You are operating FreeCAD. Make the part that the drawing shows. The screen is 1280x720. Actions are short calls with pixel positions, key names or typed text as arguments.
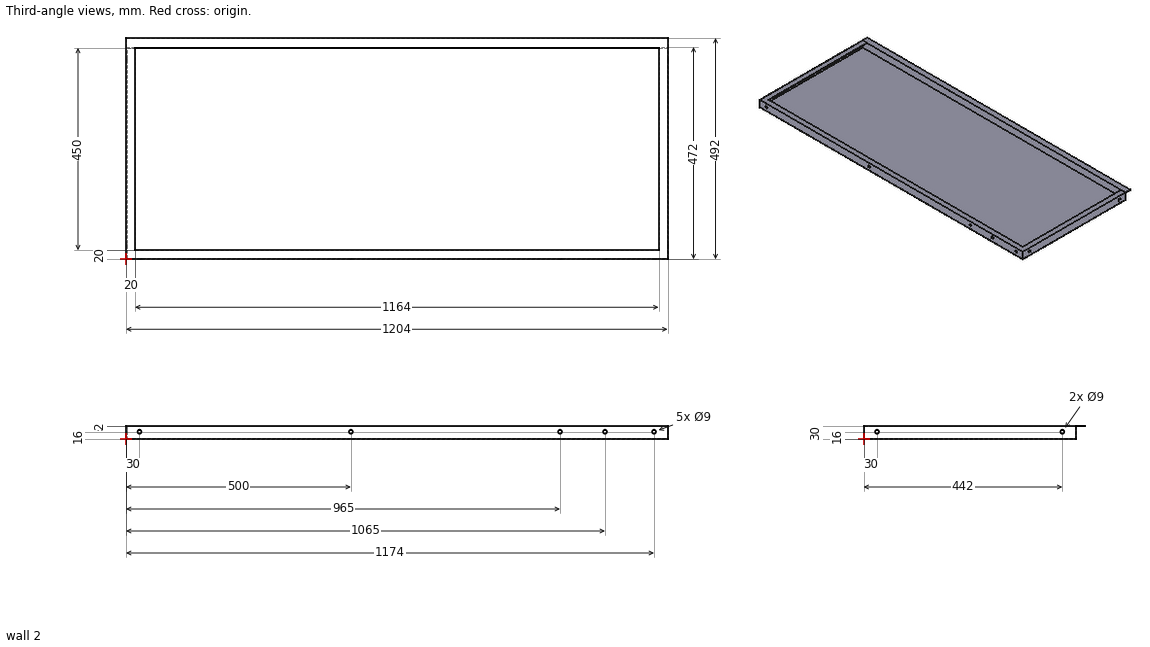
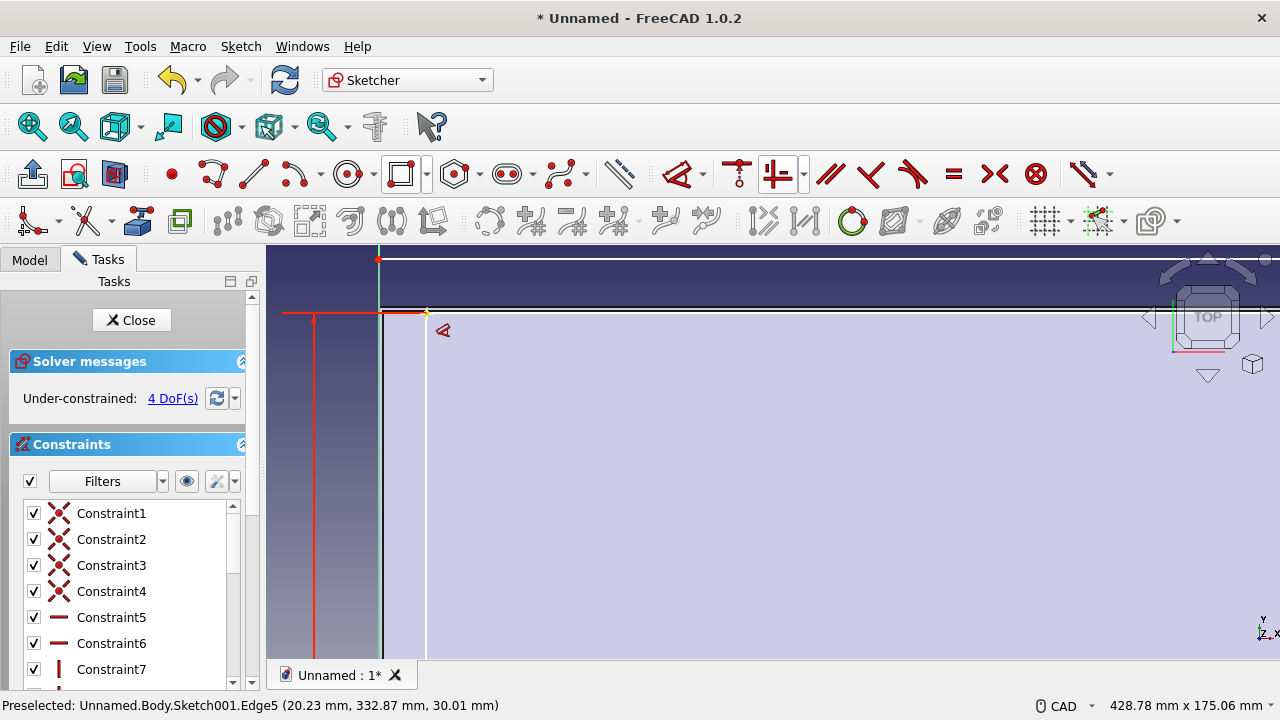
click(426, 313)
click(403, 279)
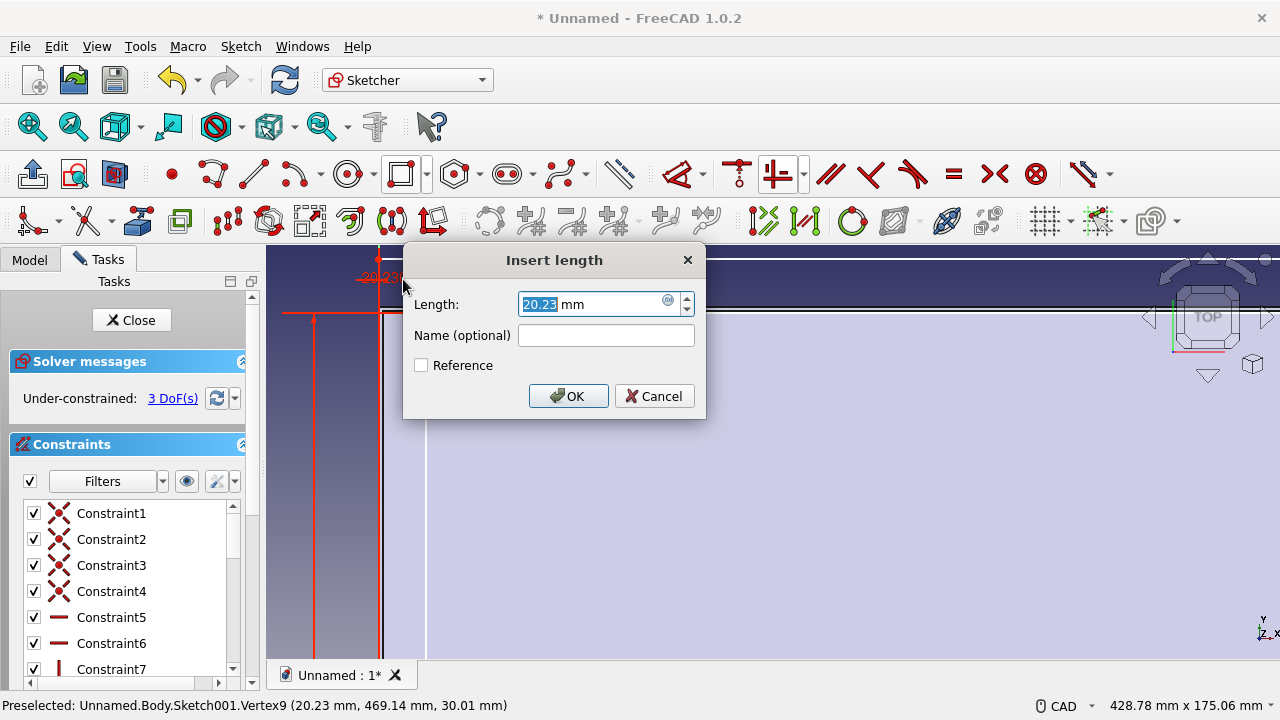
text(20)
key(Return)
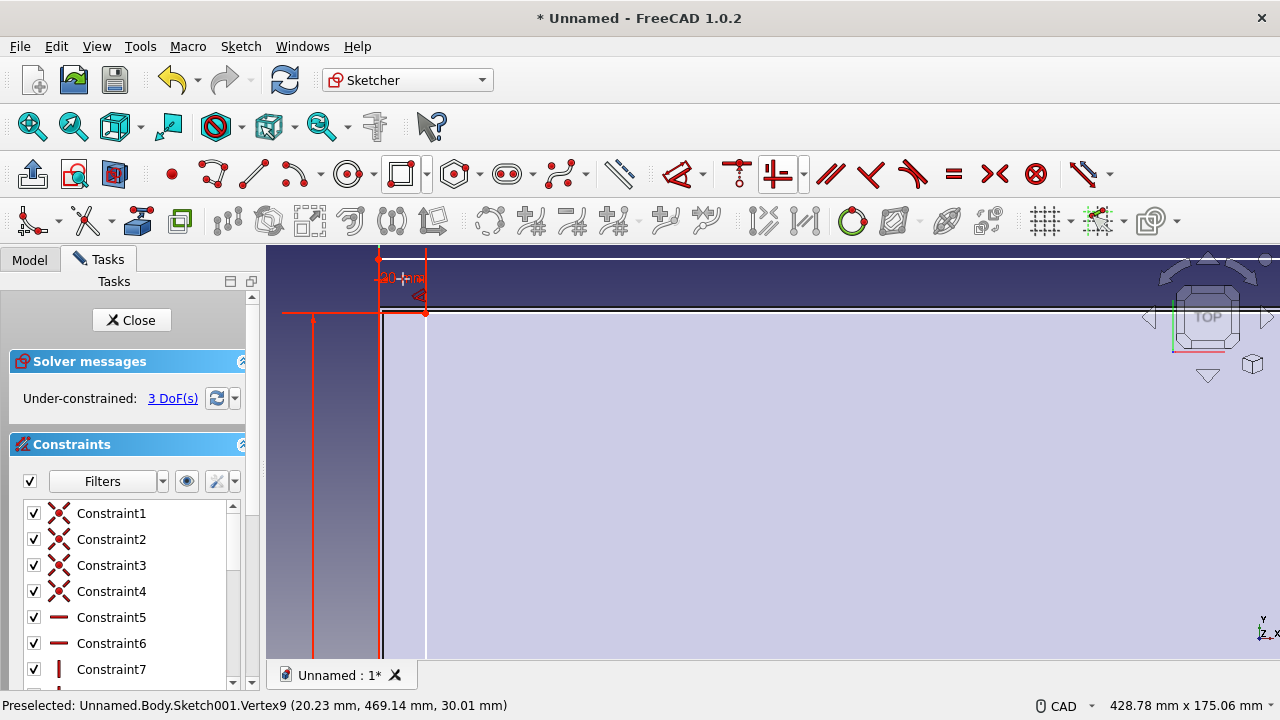
scroll(427, 354, down, 8)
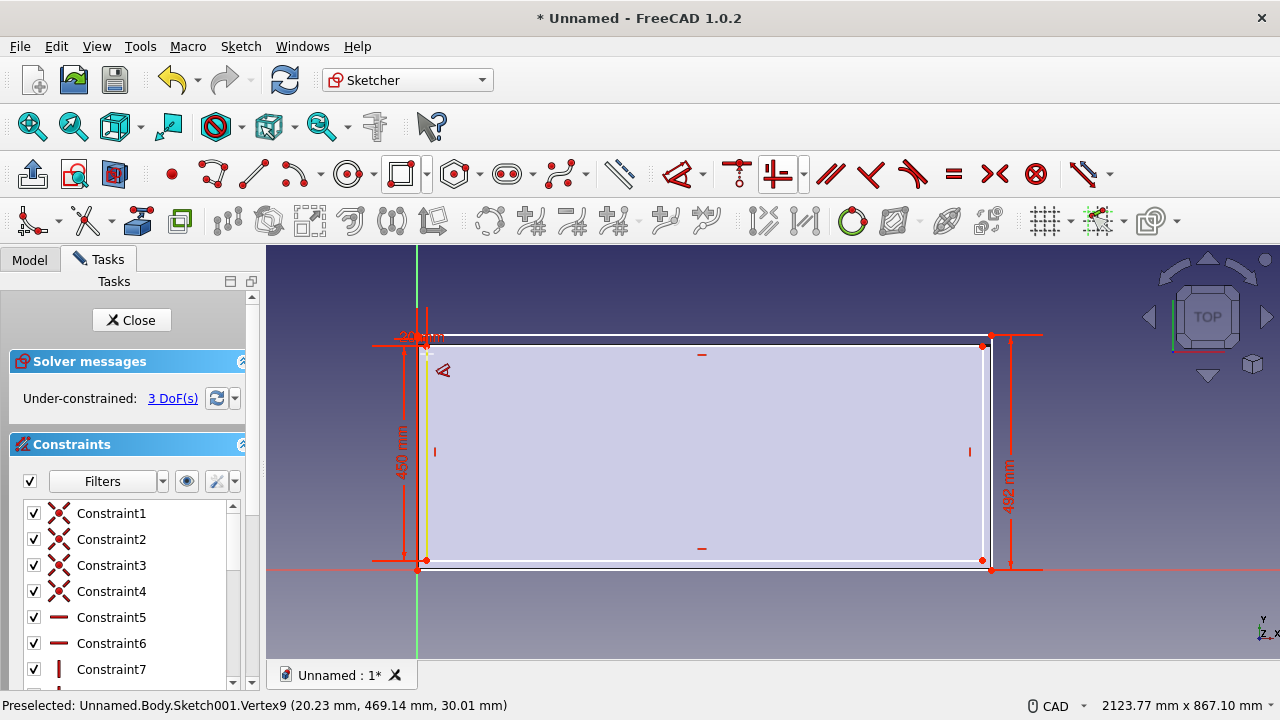
scroll(427, 561, up, 8)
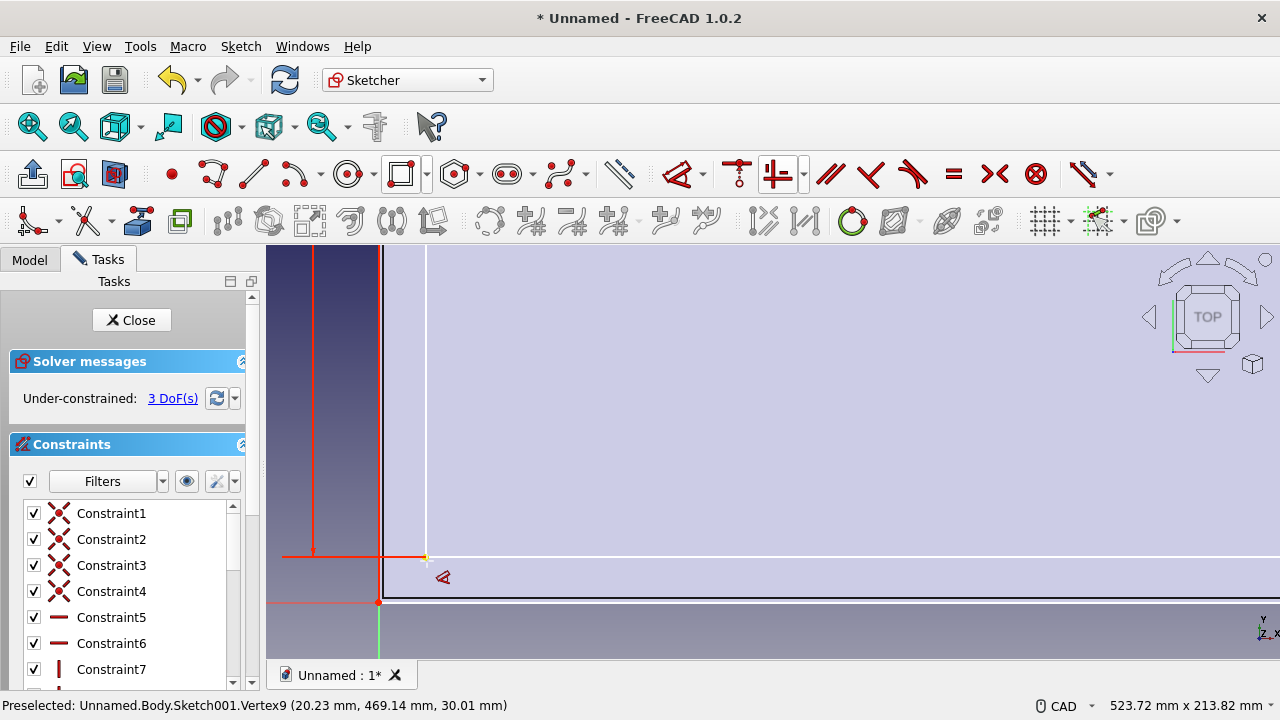
click(426, 557)
click(345, 580)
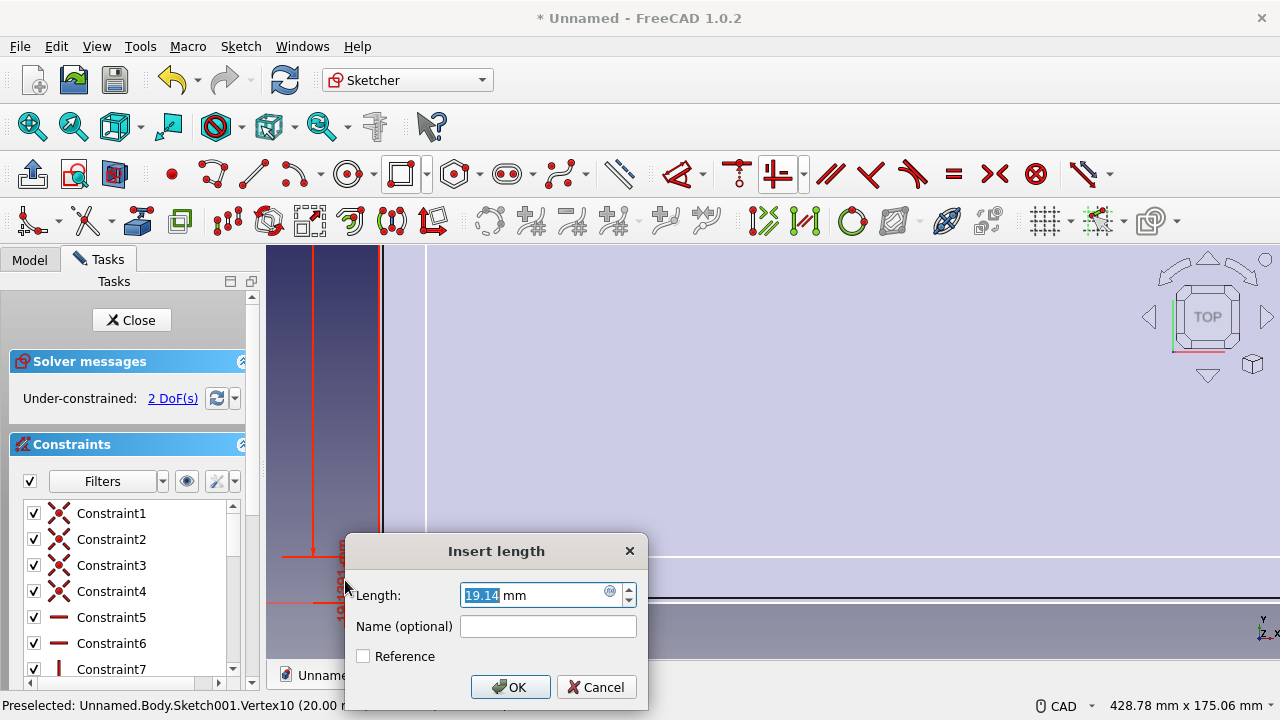
text(20)
key(Return)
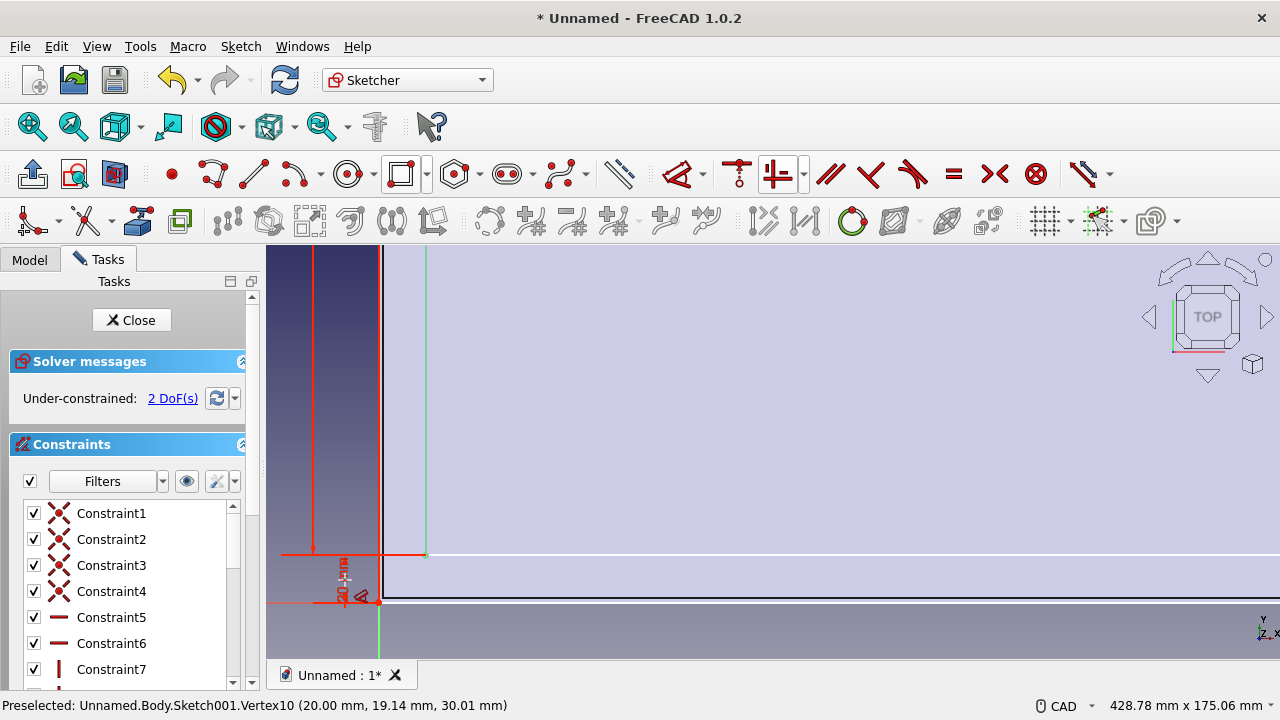
scroll(427, 561, down, 8)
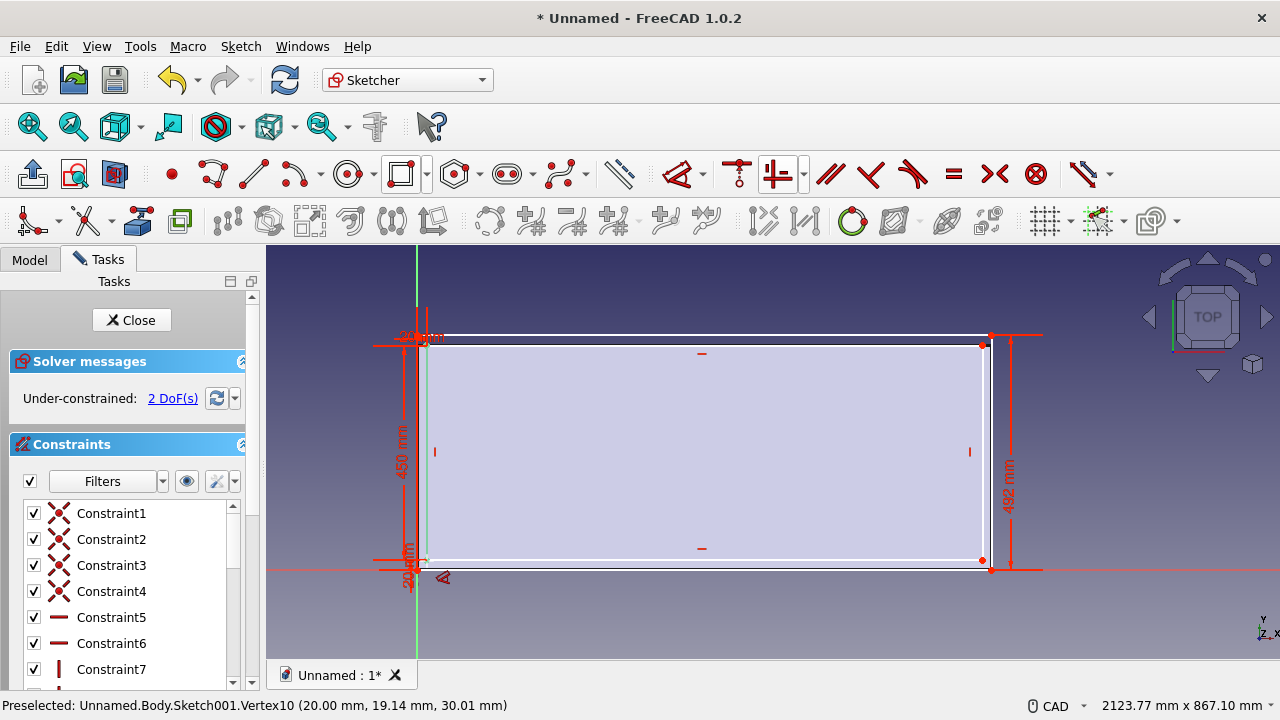
scroll(532, 570, up, 2)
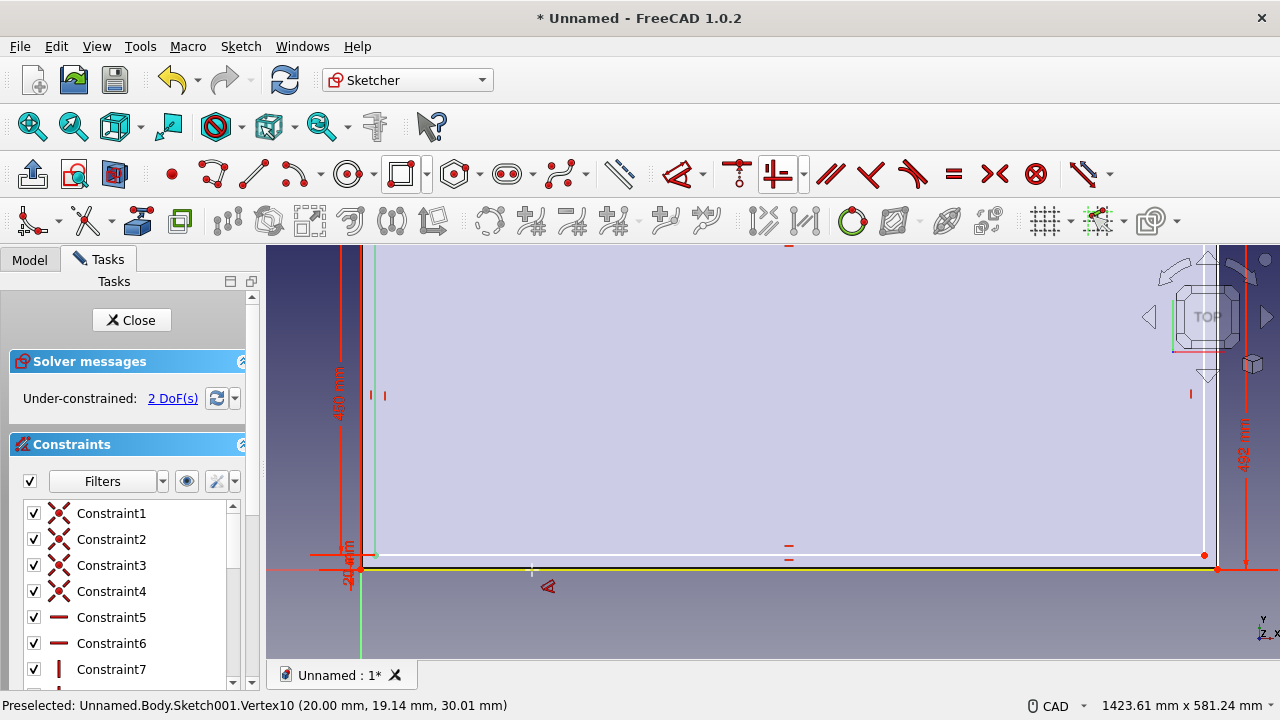
click(532, 570)
click(738, 604)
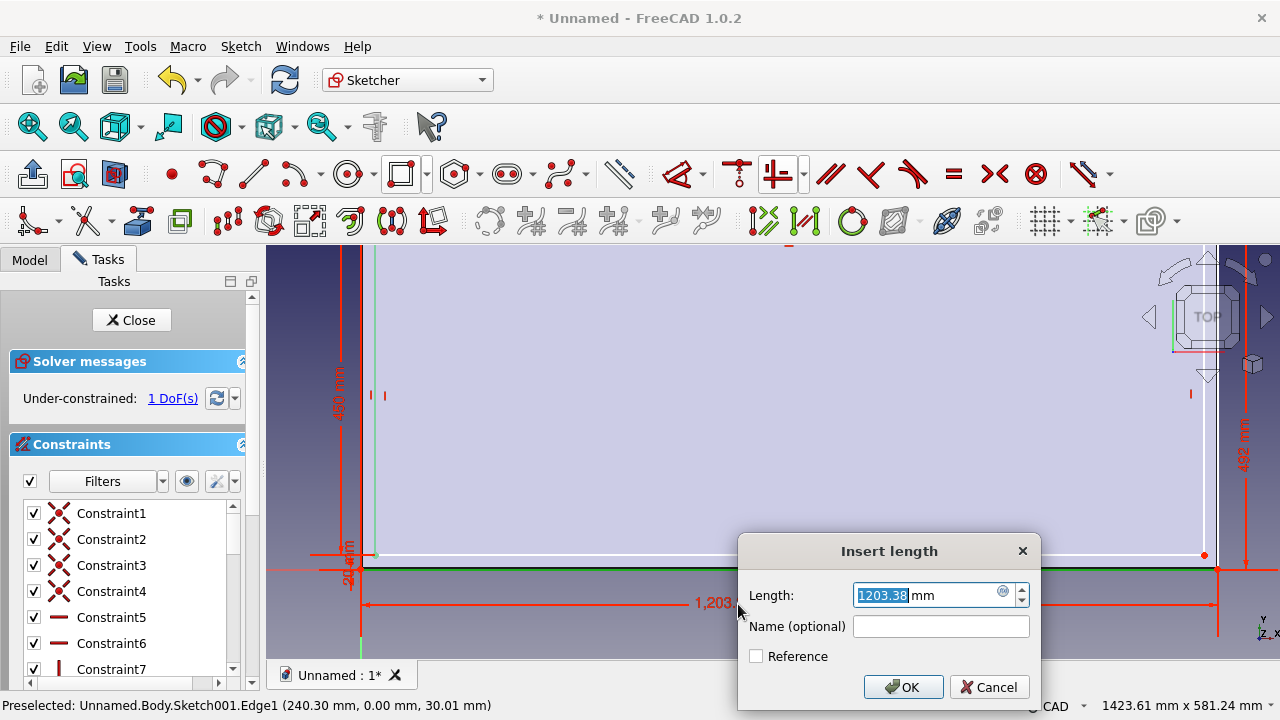
text(1204)
key(Return)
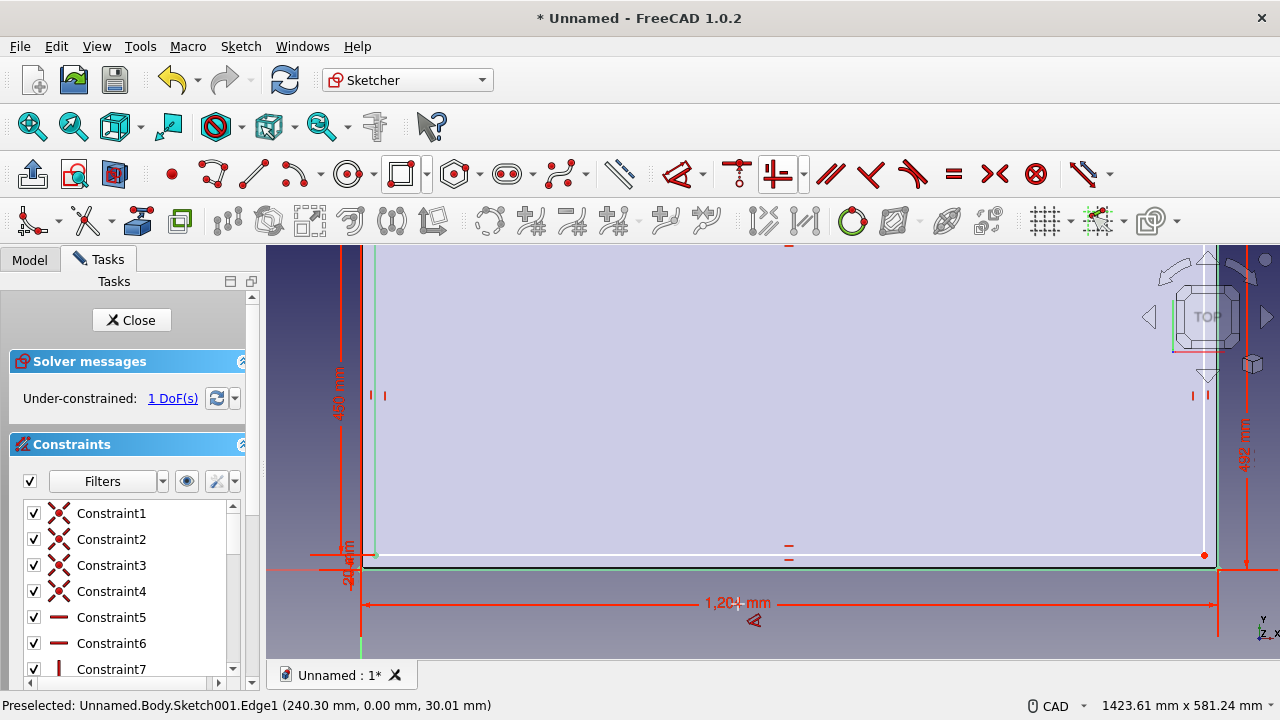
click(624, 555)
click(575, 589)